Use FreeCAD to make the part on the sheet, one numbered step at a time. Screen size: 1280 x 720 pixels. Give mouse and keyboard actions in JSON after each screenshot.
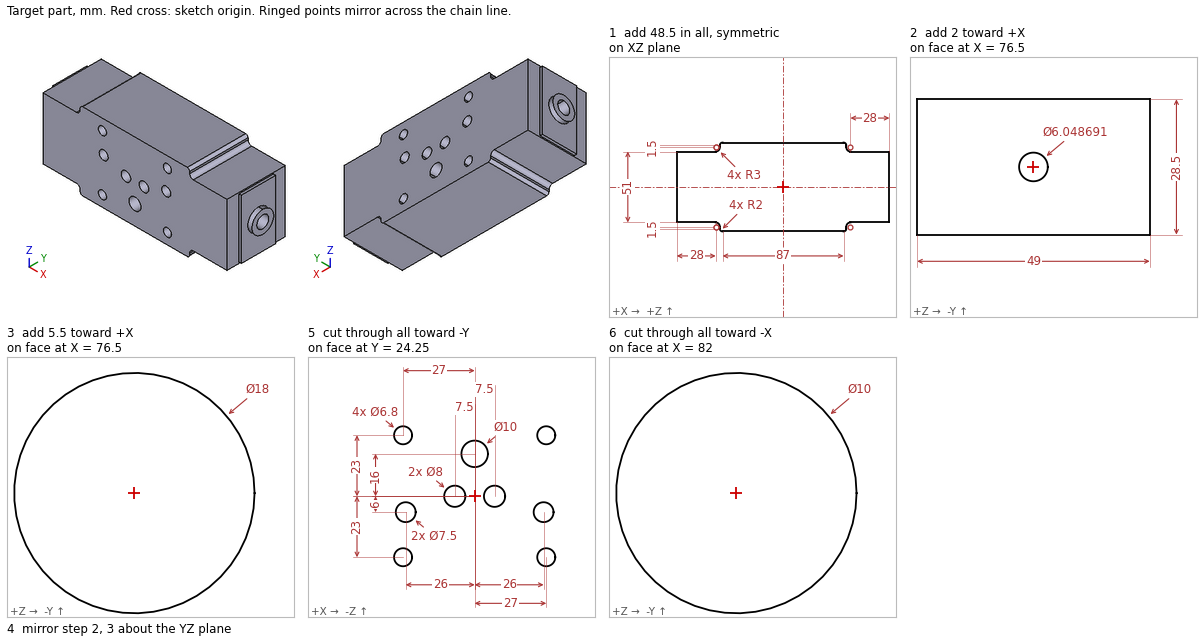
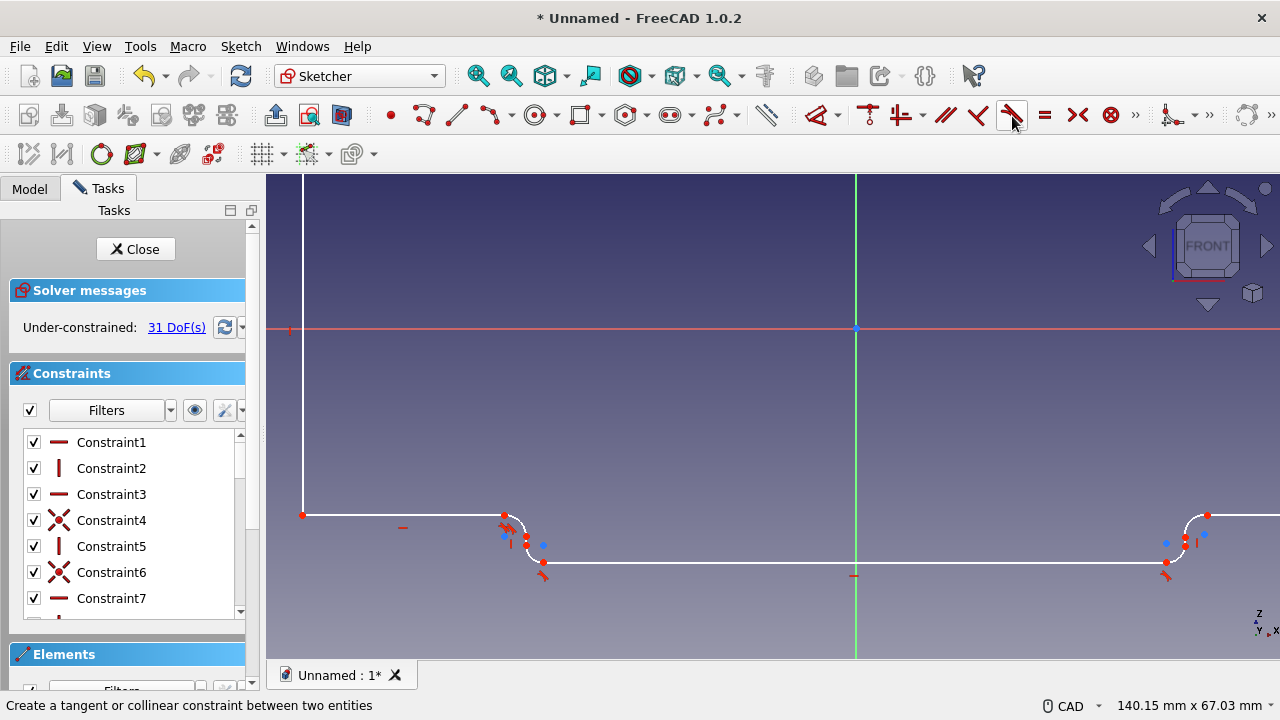
{"action": "scroll", "coordinate": [520, 523], "scroll_direction": "down", "scroll_amount": 3}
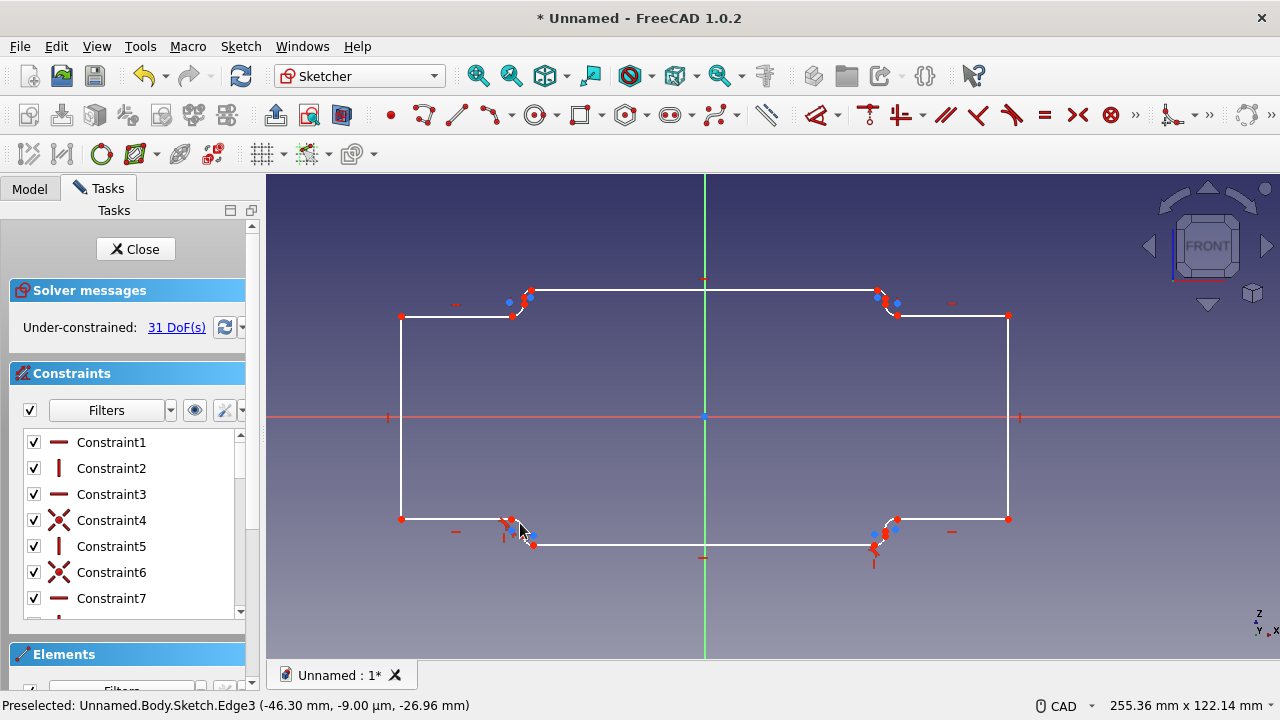
{"action": "left_click", "coordinate": [434, 317]}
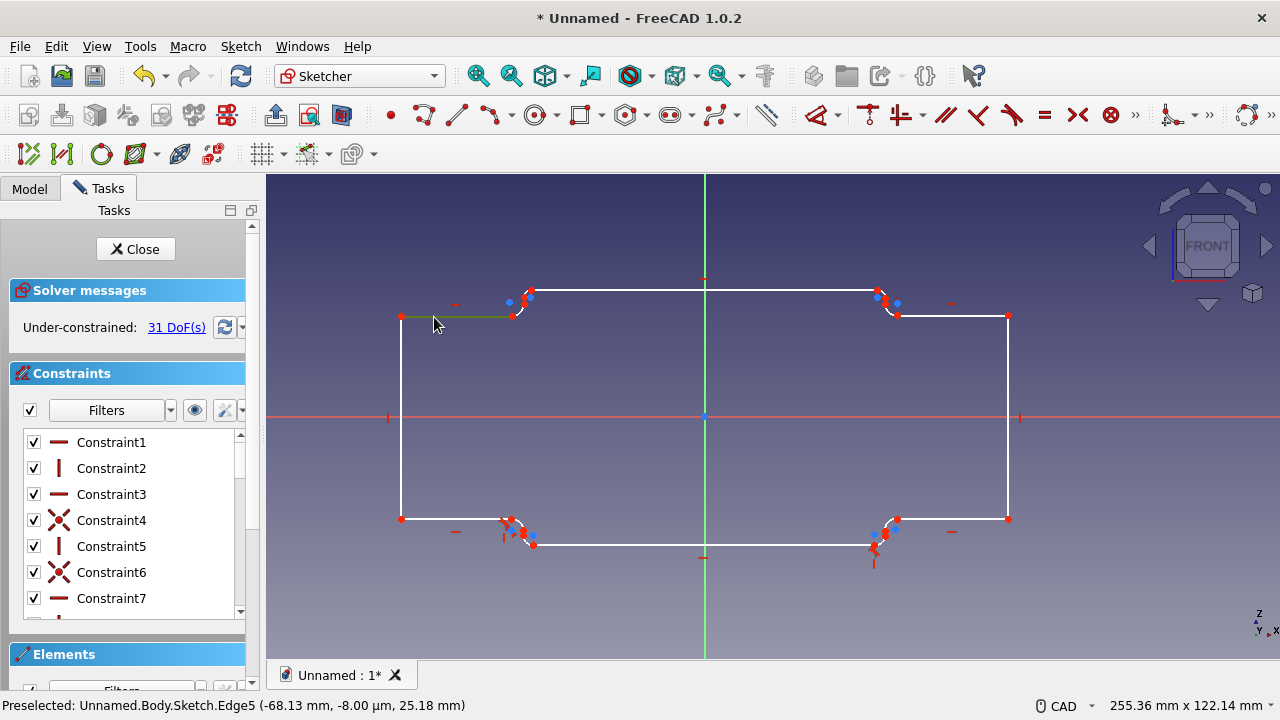
{"action": "scroll", "coordinate": [520, 313], "scroll_direction": "up", "scroll_amount": 3}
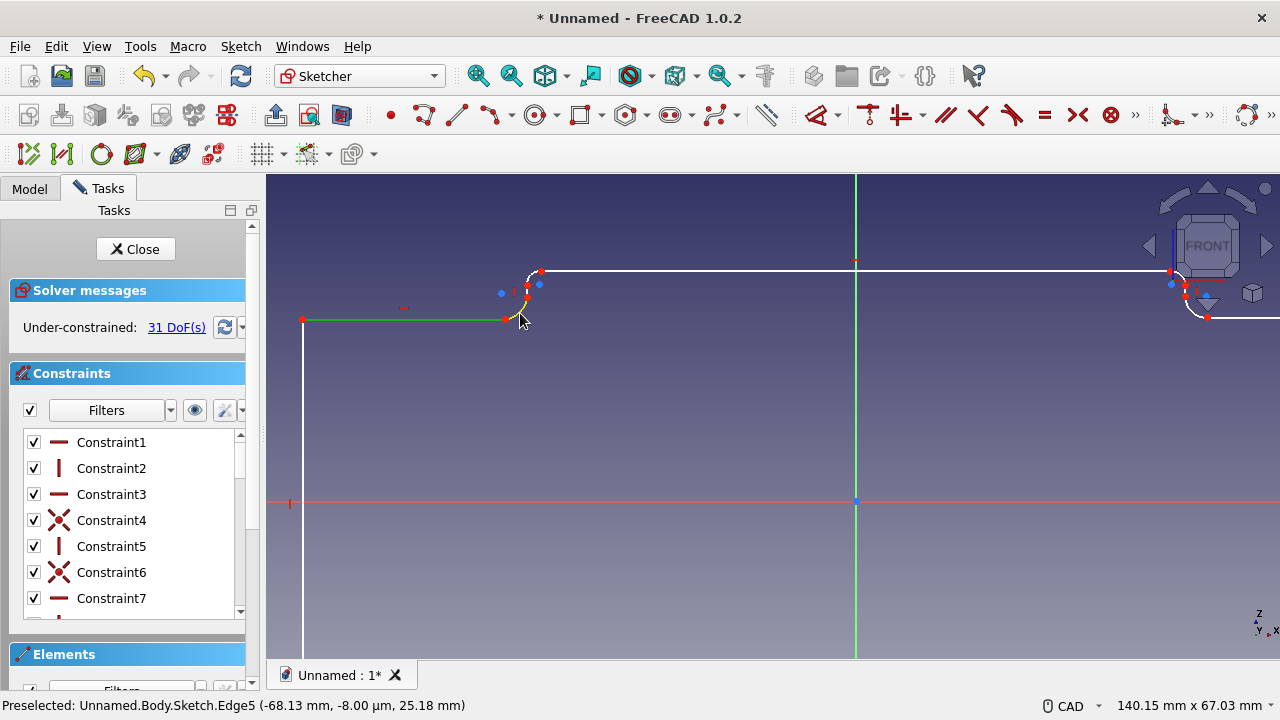
{"action": "left_click", "coordinate": [520, 312]}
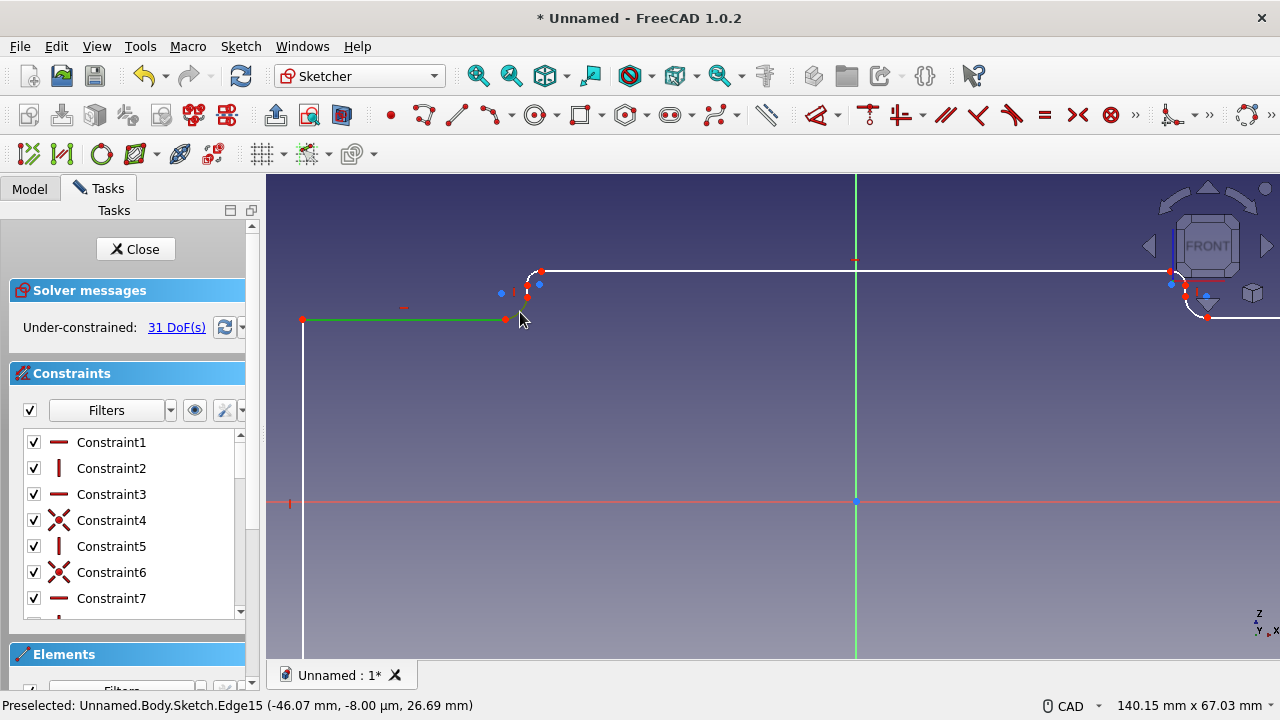
{"action": "left_click", "coordinate": [1012, 116]}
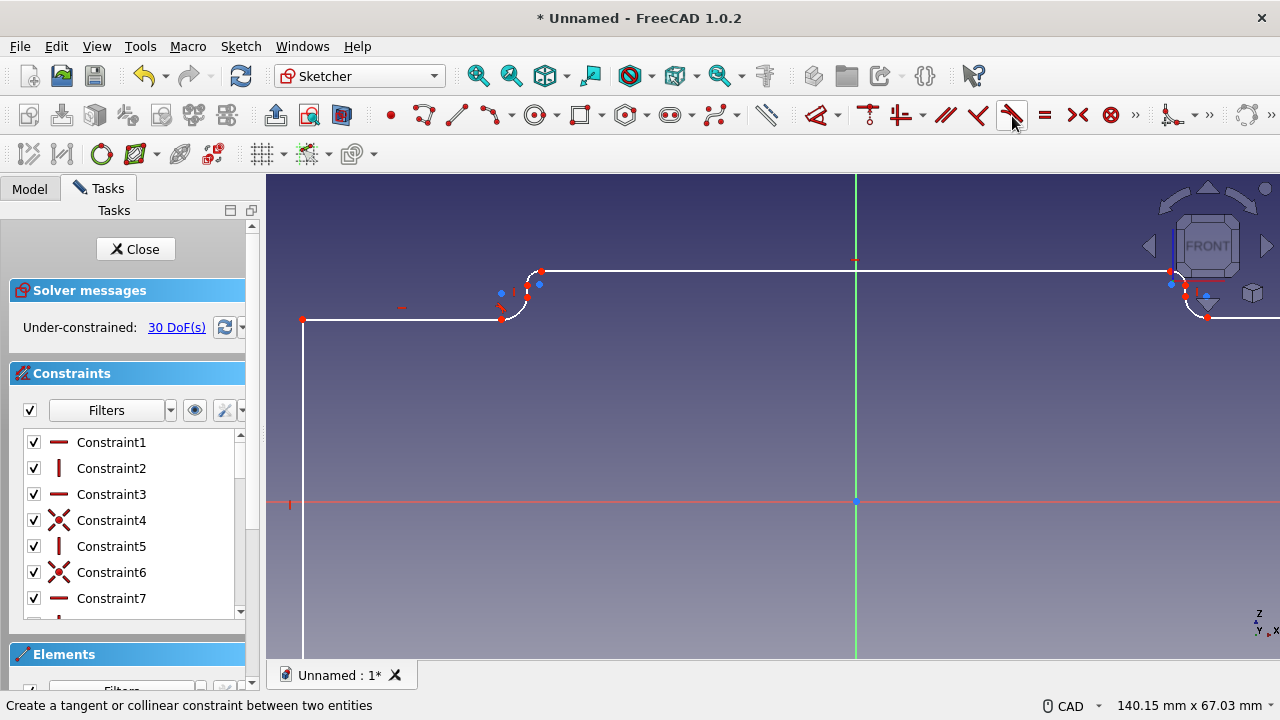
{"action": "scroll", "coordinate": [527, 292], "scroll_direction": "up", "scroll_amount": 4}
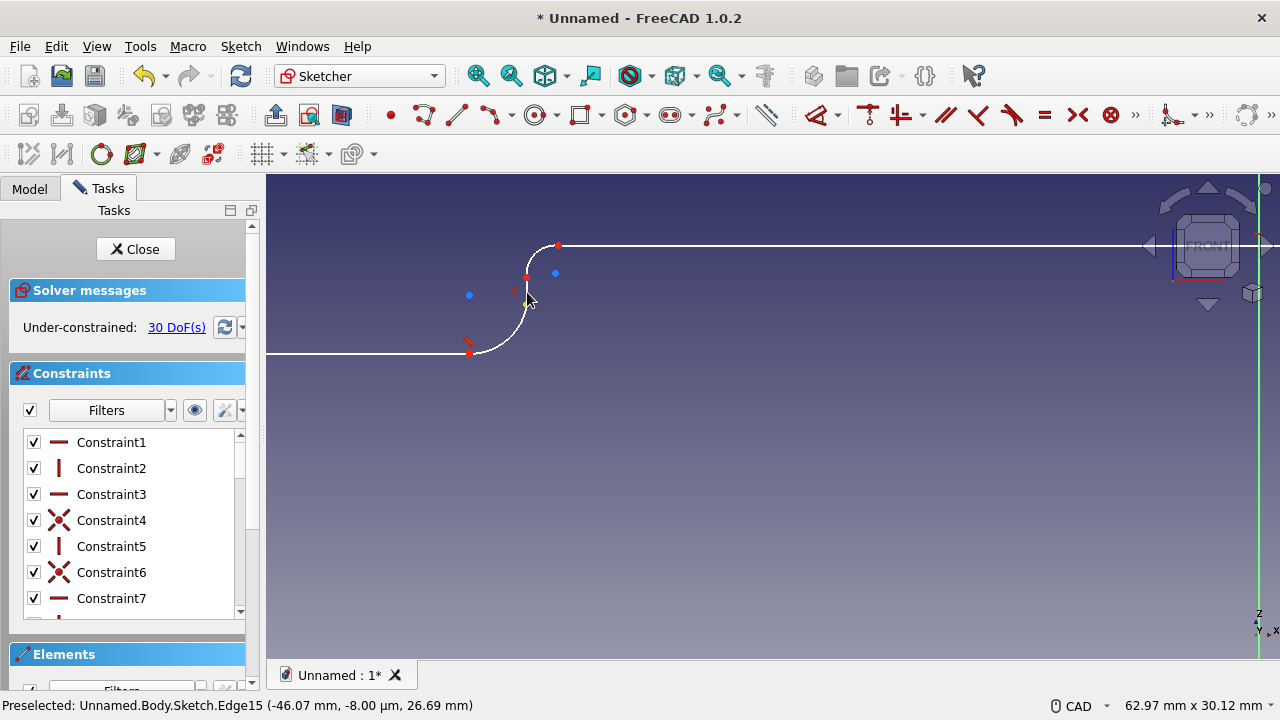
{"action": "left_click", "coordinate": [527, 291]}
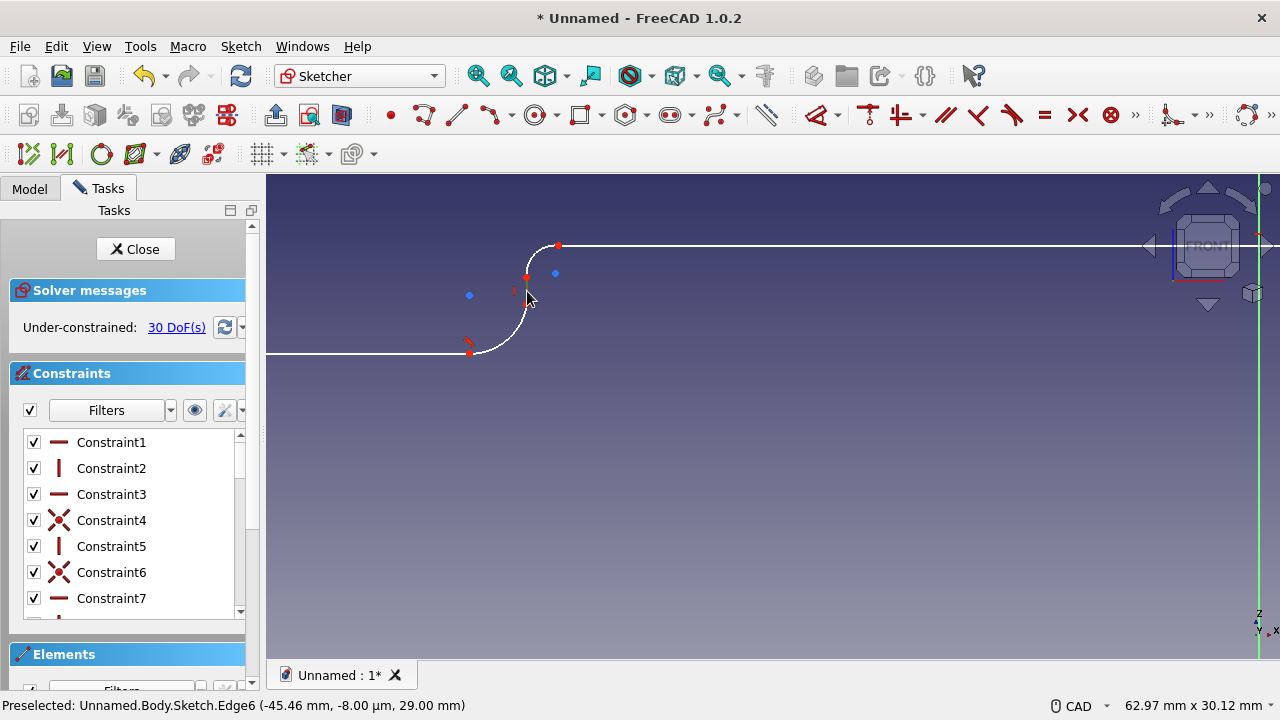
{"action": "left_click", "coordinate": [493, 349]}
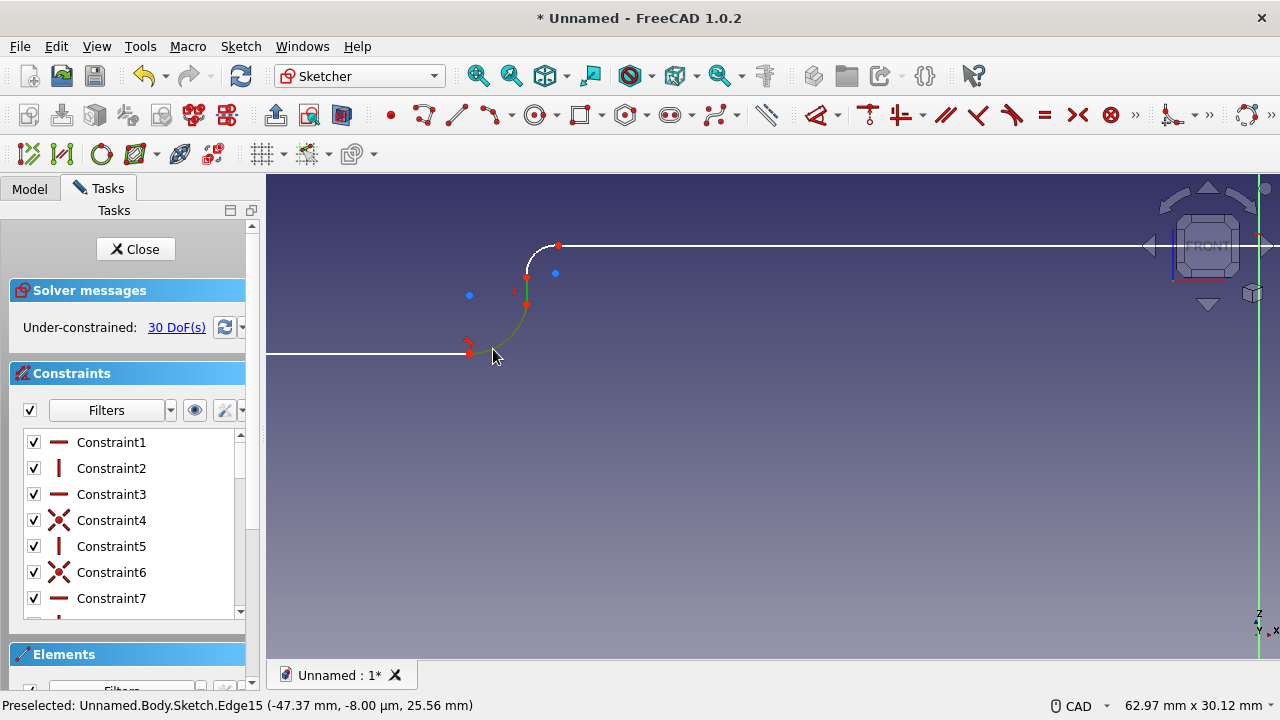
{"action": "left_click", "coordinate": [1012, 116]}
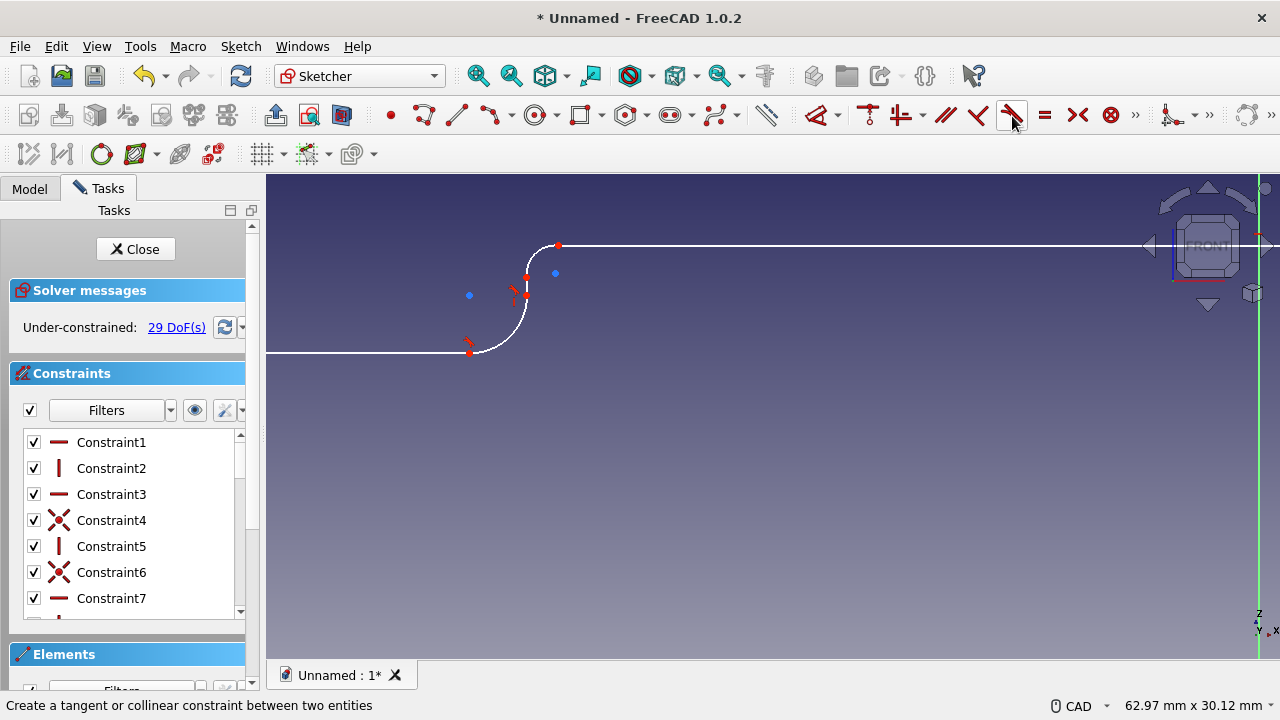
{"action": "scroll", "coordinate": [527, 286], "scroll_direction": "up", "scroll_amount": 2}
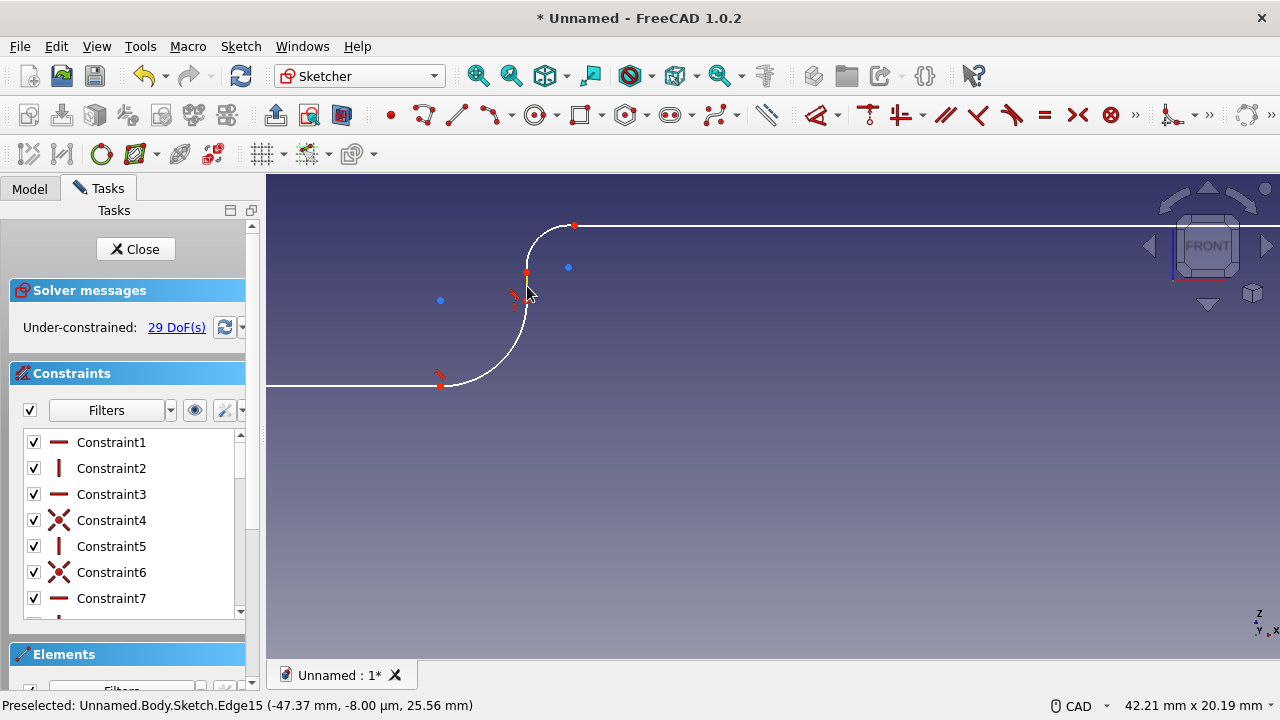
{"action": "left_click", "coordinate": [527, 286]}